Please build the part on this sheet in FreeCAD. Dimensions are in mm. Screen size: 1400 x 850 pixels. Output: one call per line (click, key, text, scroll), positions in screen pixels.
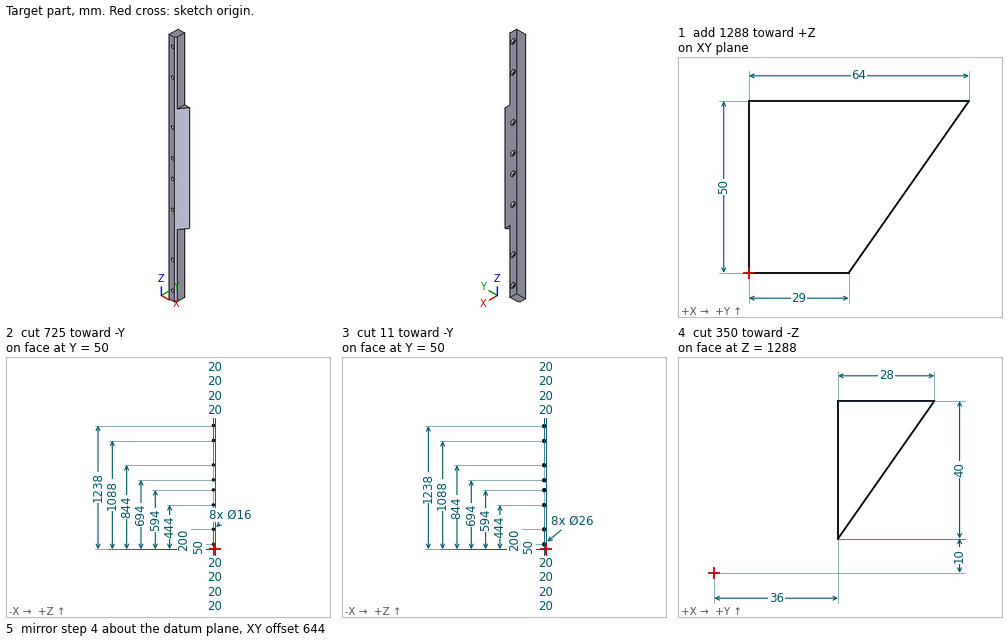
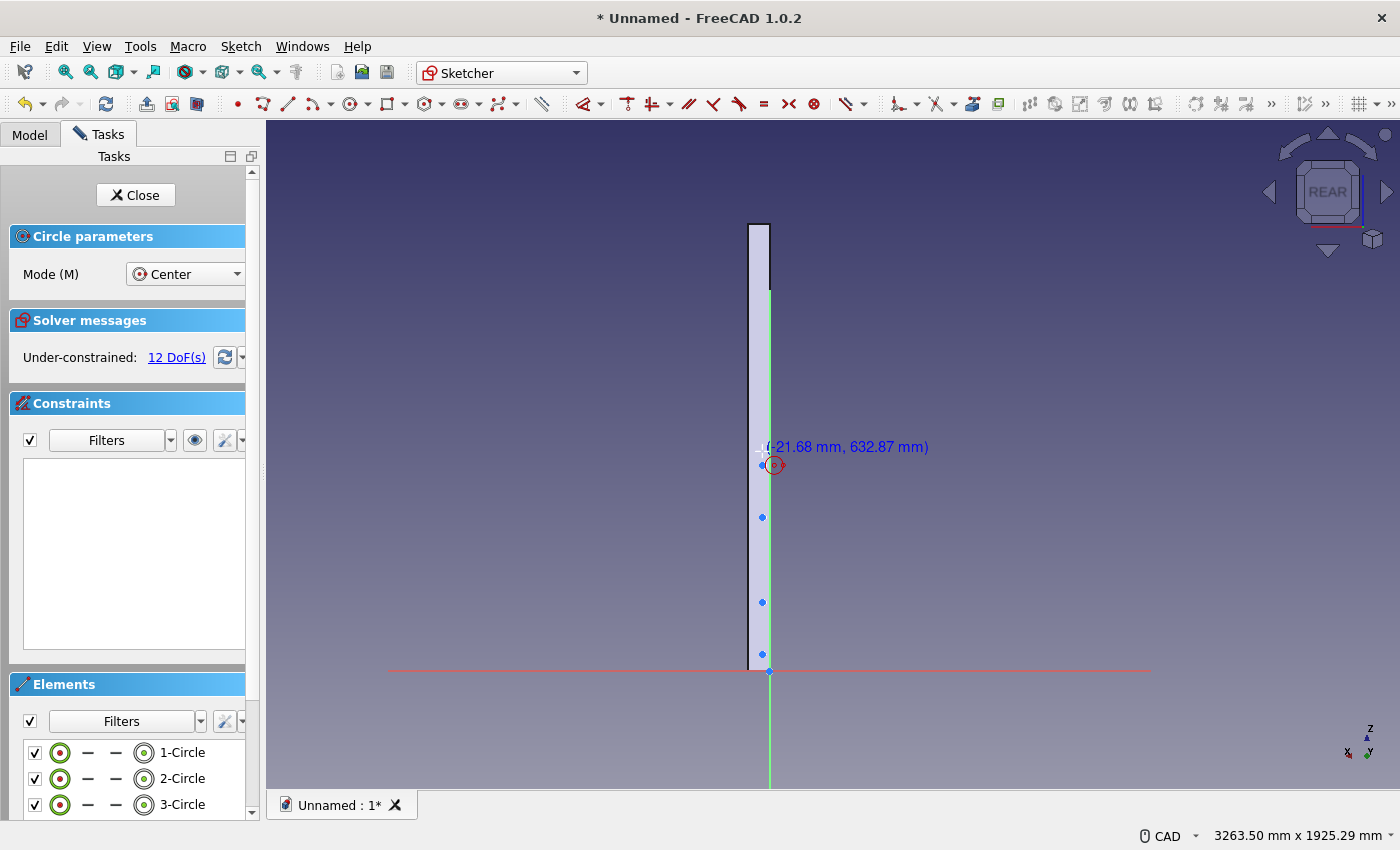
scroll(763, 430, up, 5)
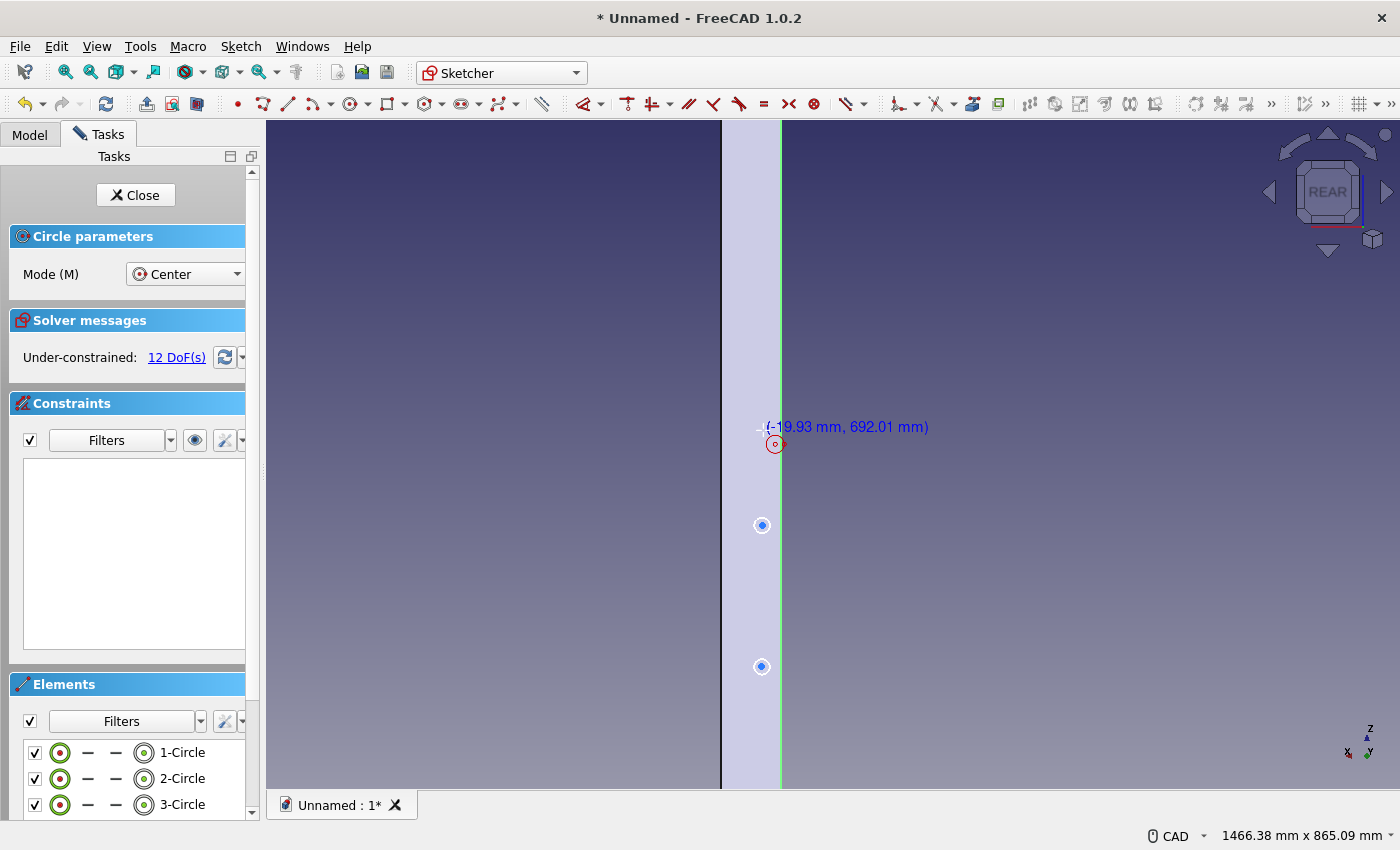
click(762, 430)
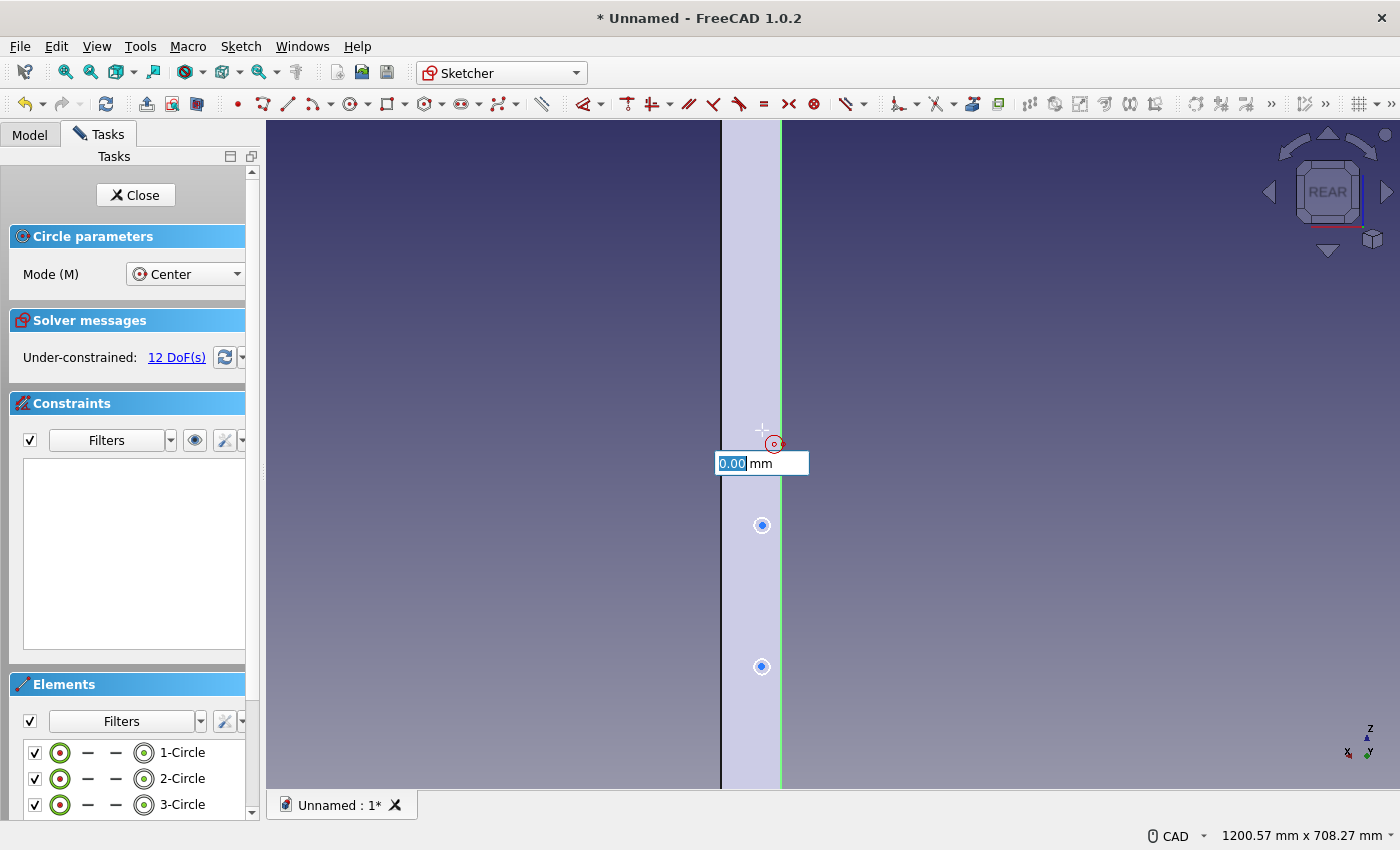
scroll(757, 425, up, 4)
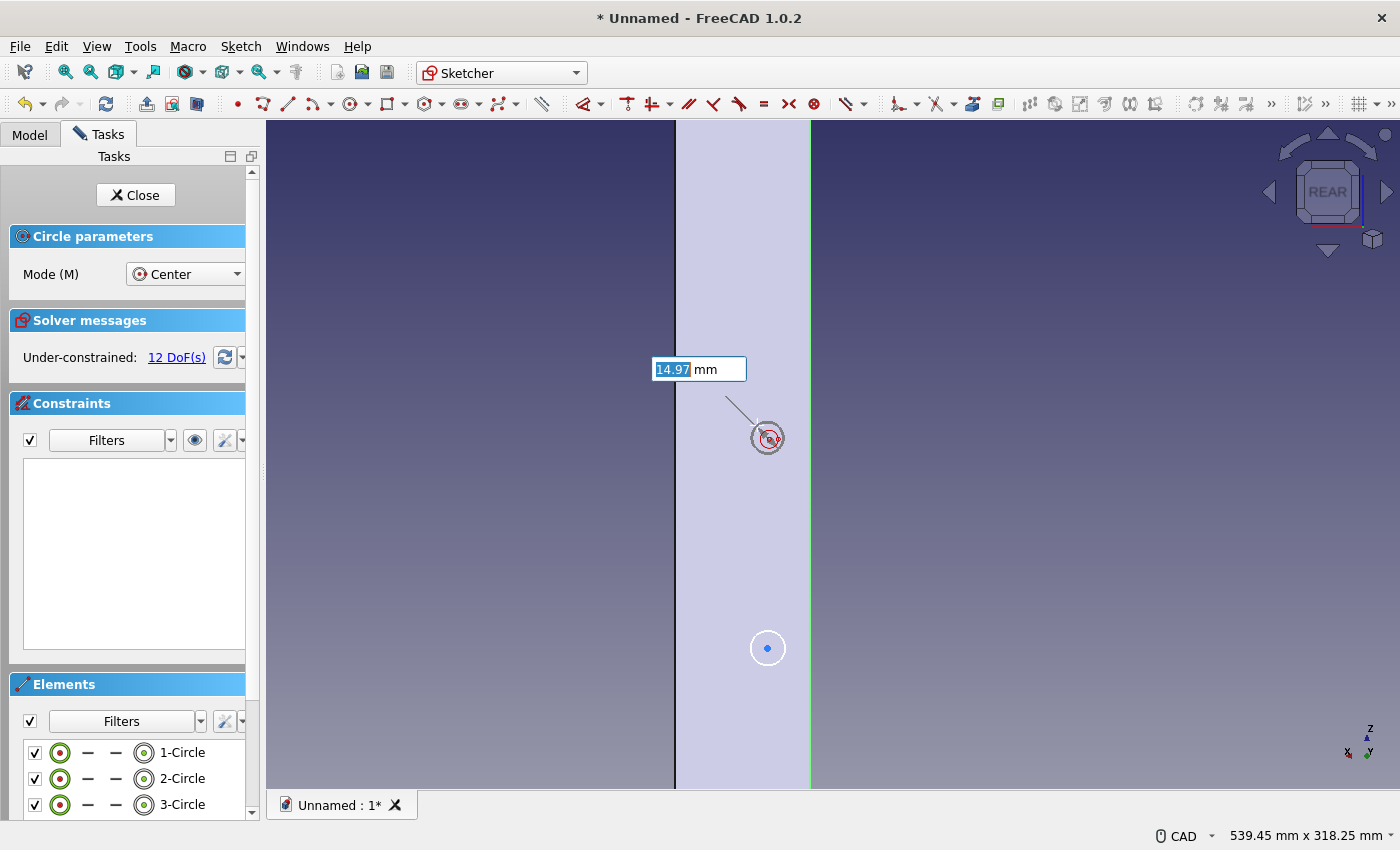
click(756, 424)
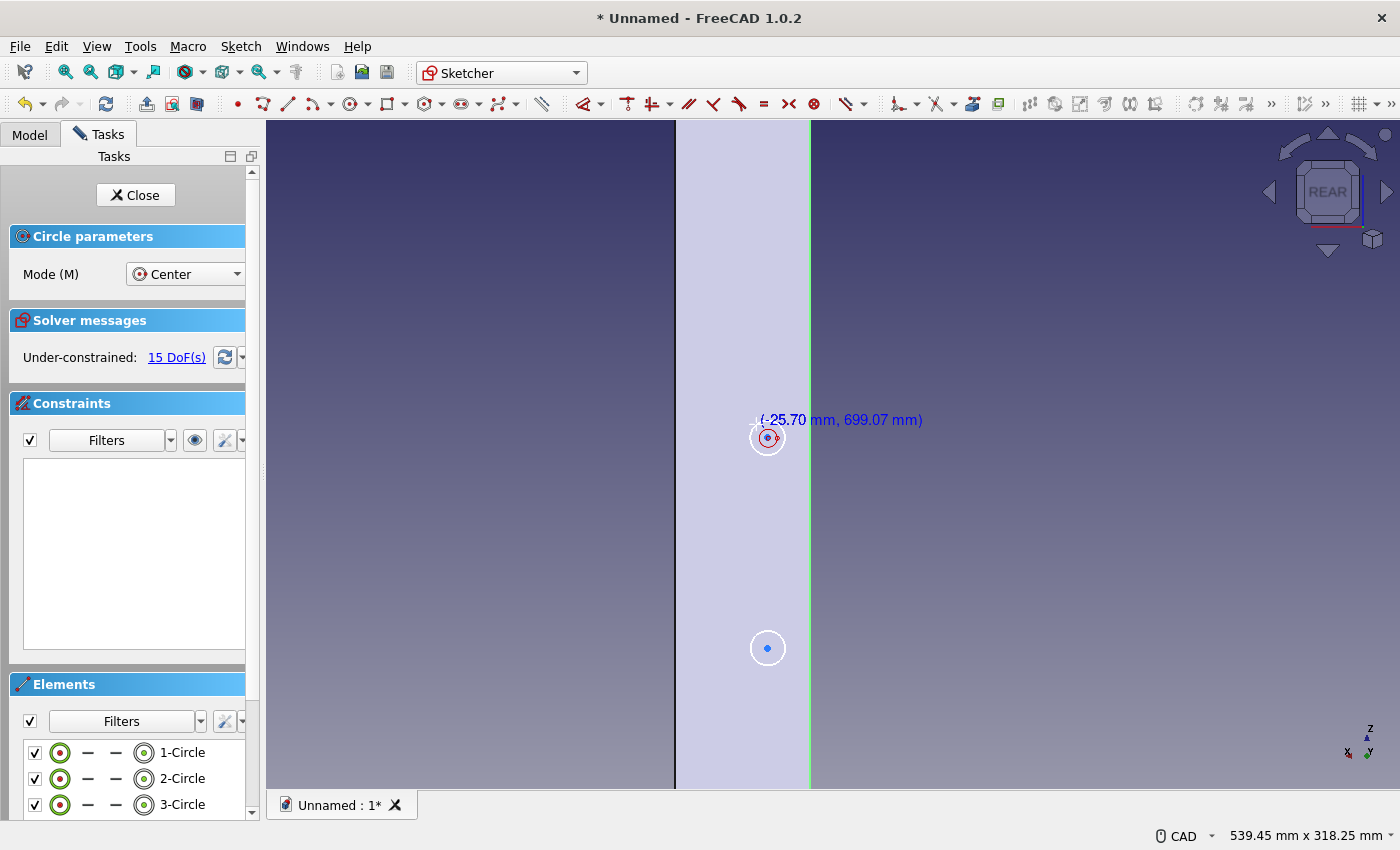
scroll(761, 429, down, 9)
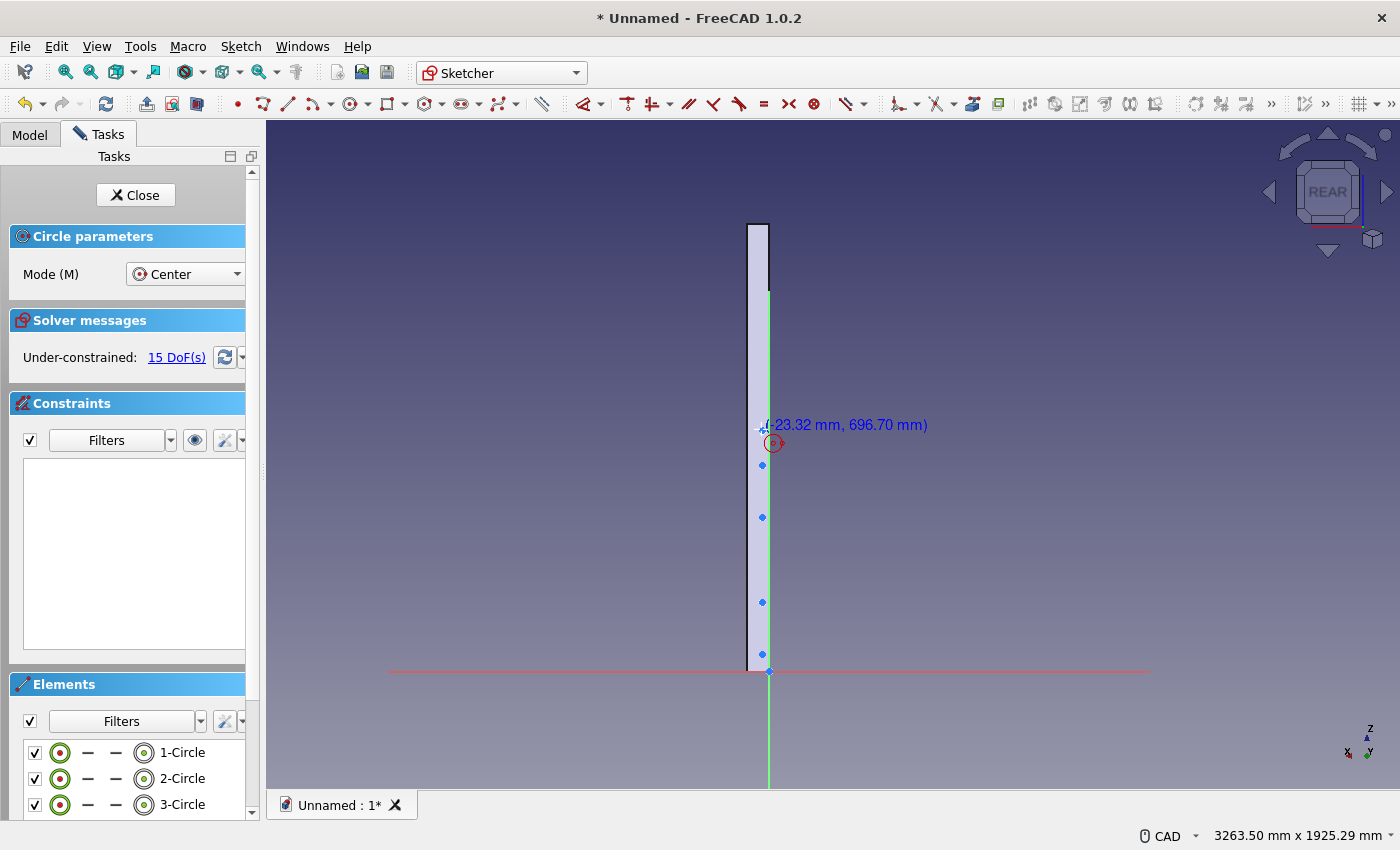
scroll(763, 378, up, 11)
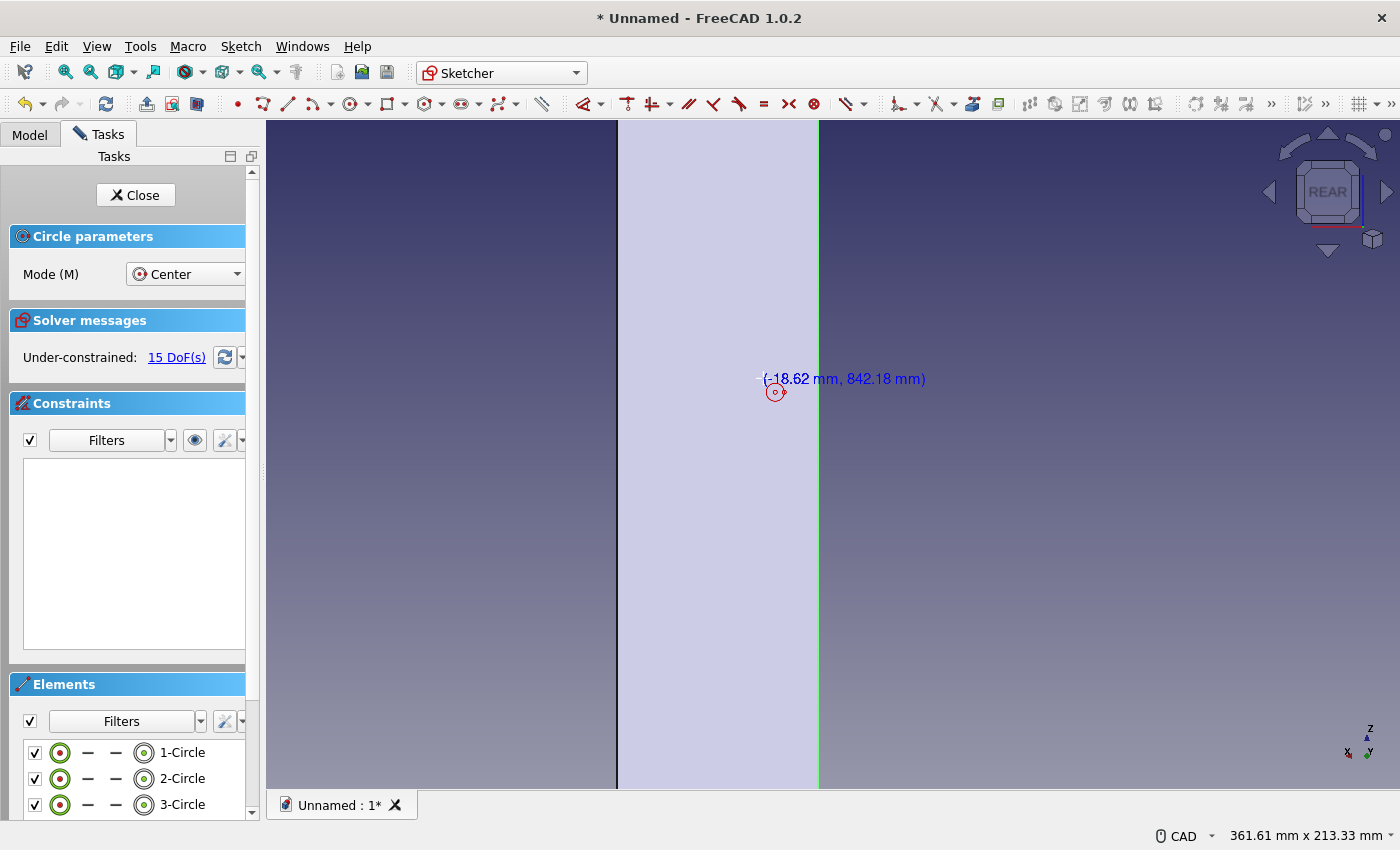
scroll(763, 378, down, 11)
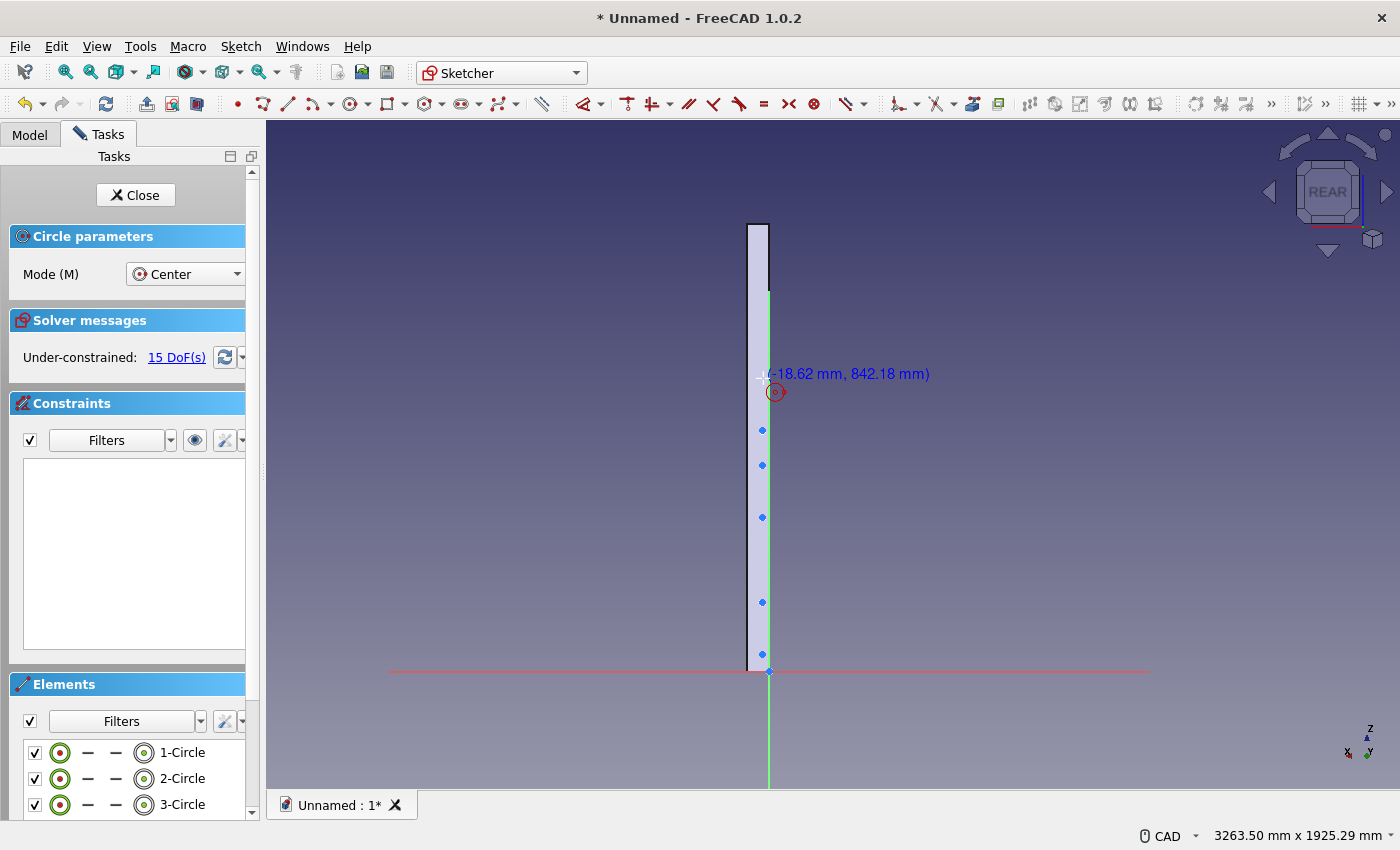
scroll(763, 378, up, 5)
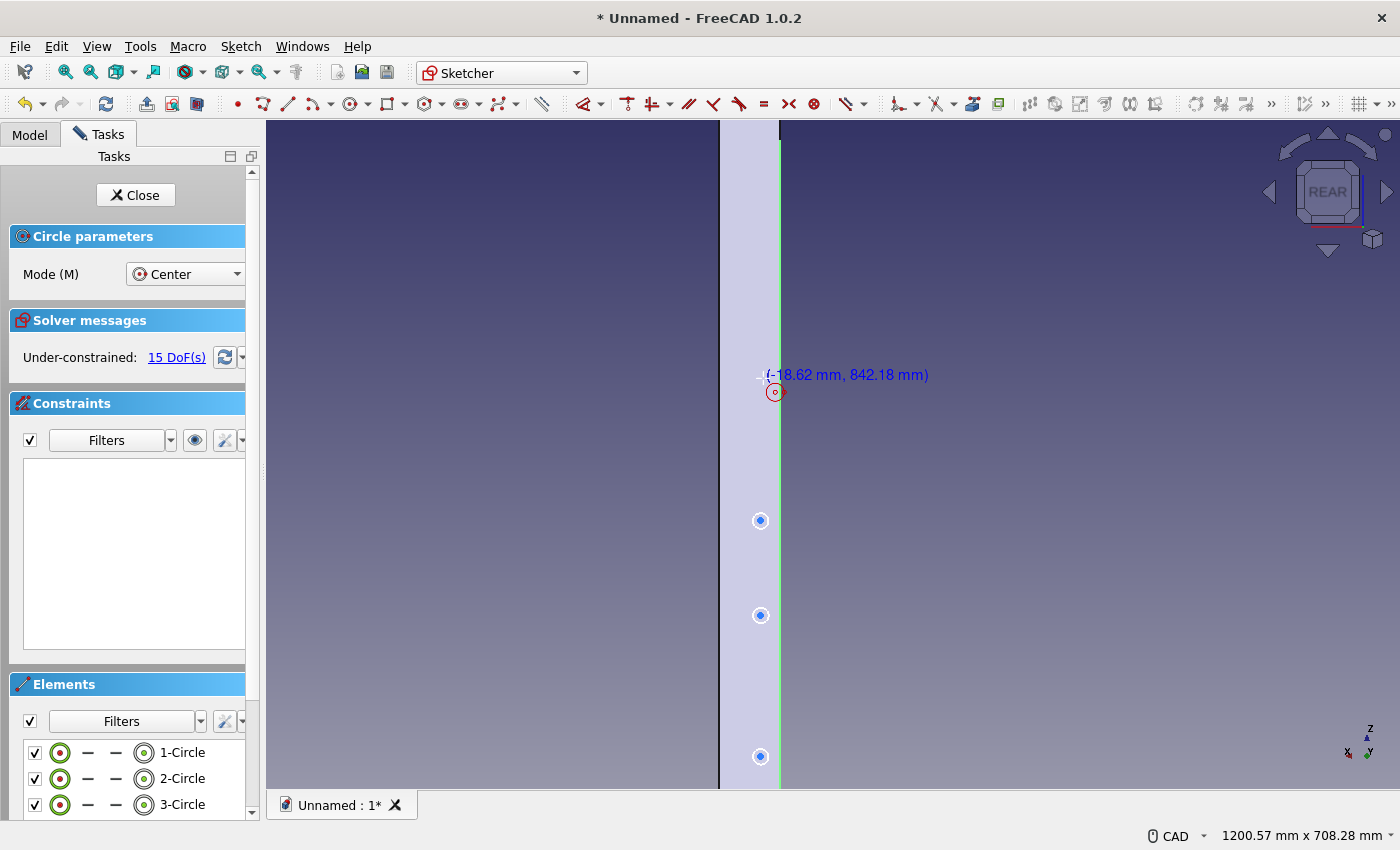
click(761, 378)